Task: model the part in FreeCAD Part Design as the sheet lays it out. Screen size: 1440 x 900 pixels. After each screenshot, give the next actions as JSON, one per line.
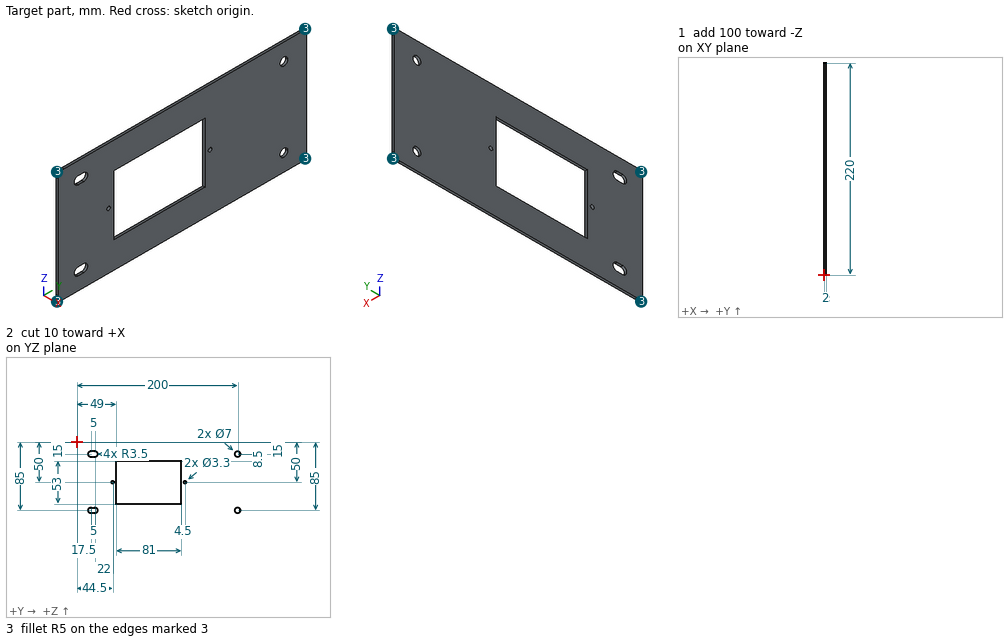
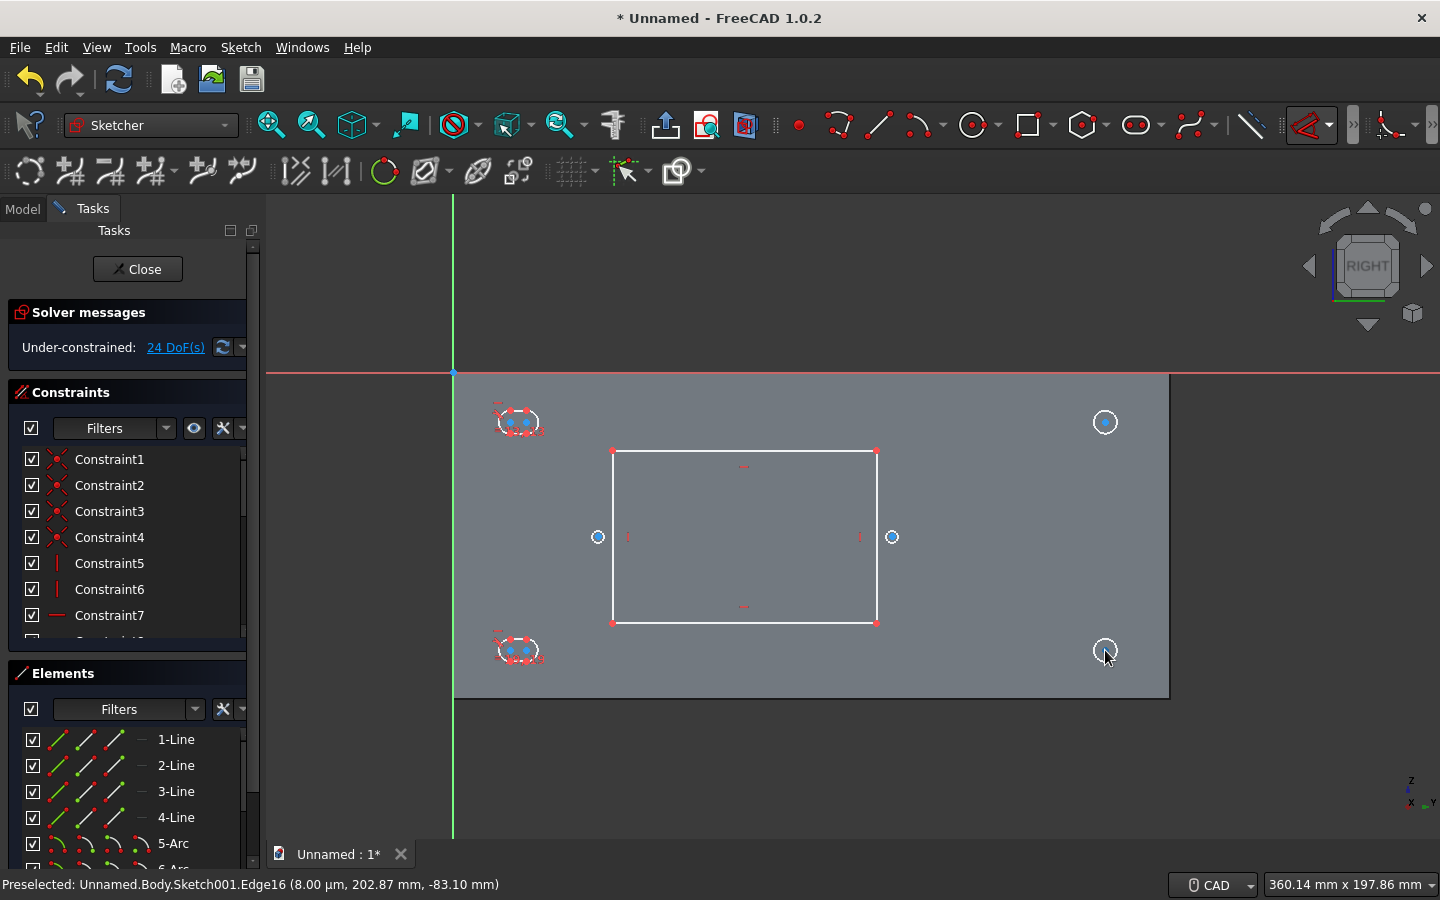
{"action": "scroll", "coordinate": [501, 415], "scroll_direction": "up", "scroll_amount": 2}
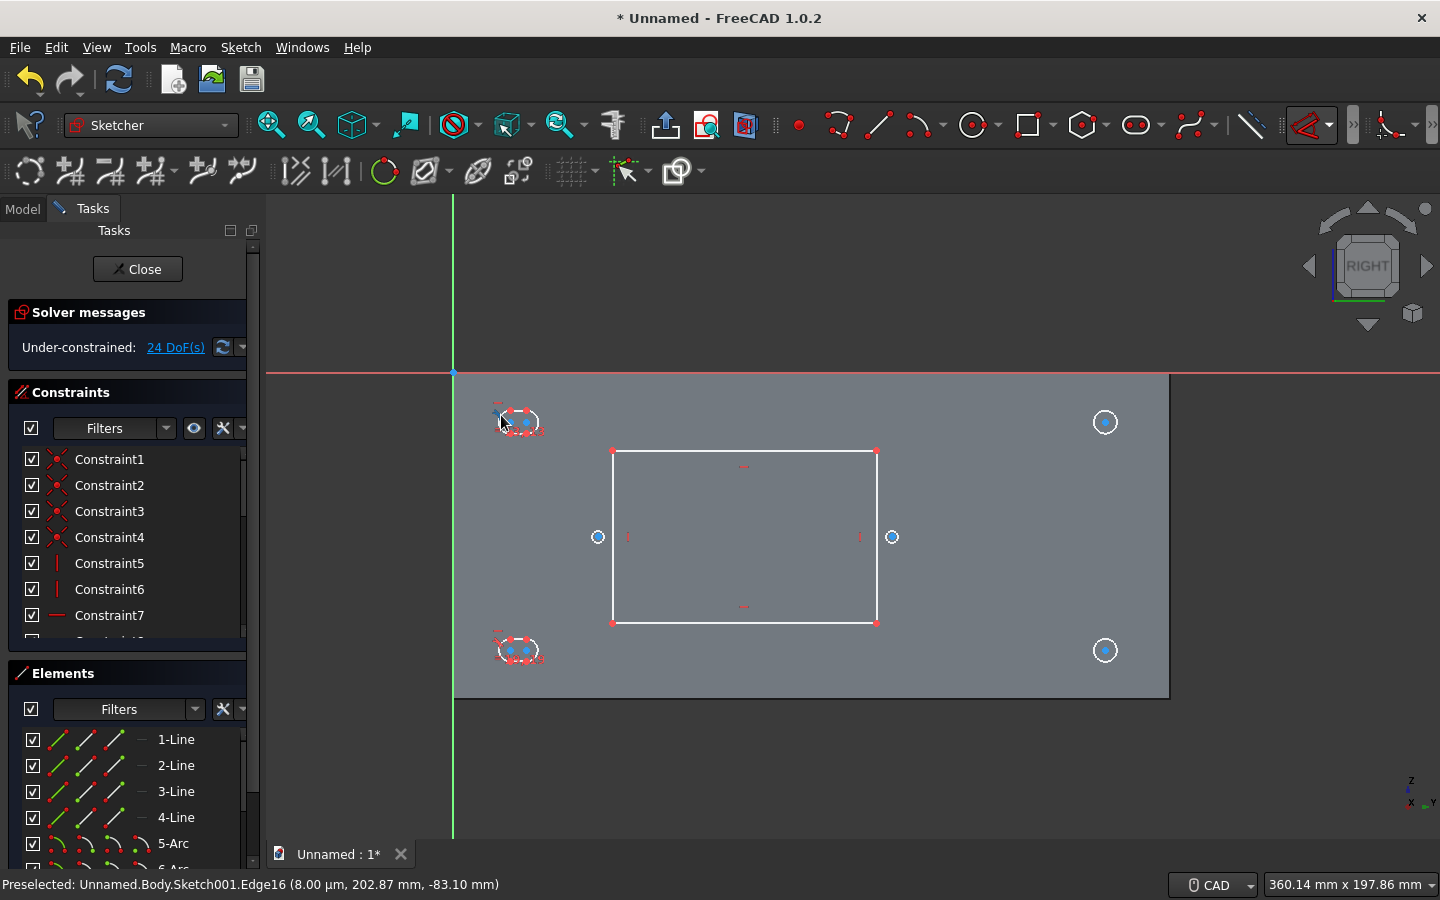
{"action": "left_click", "coordinate": [501, 415]}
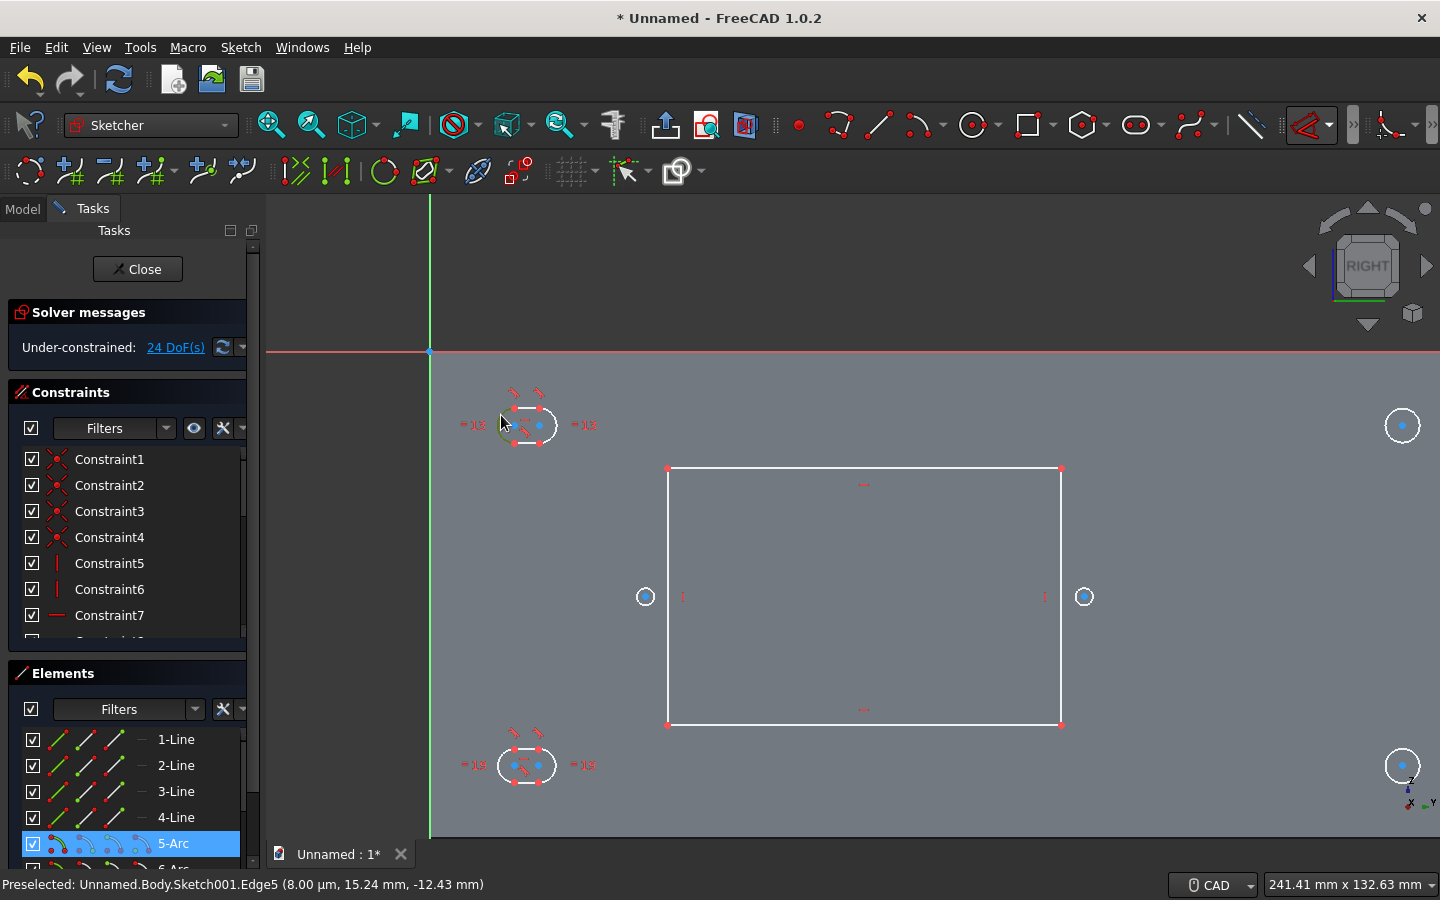
{"action": "left_click", "coordinate": [501, 756]}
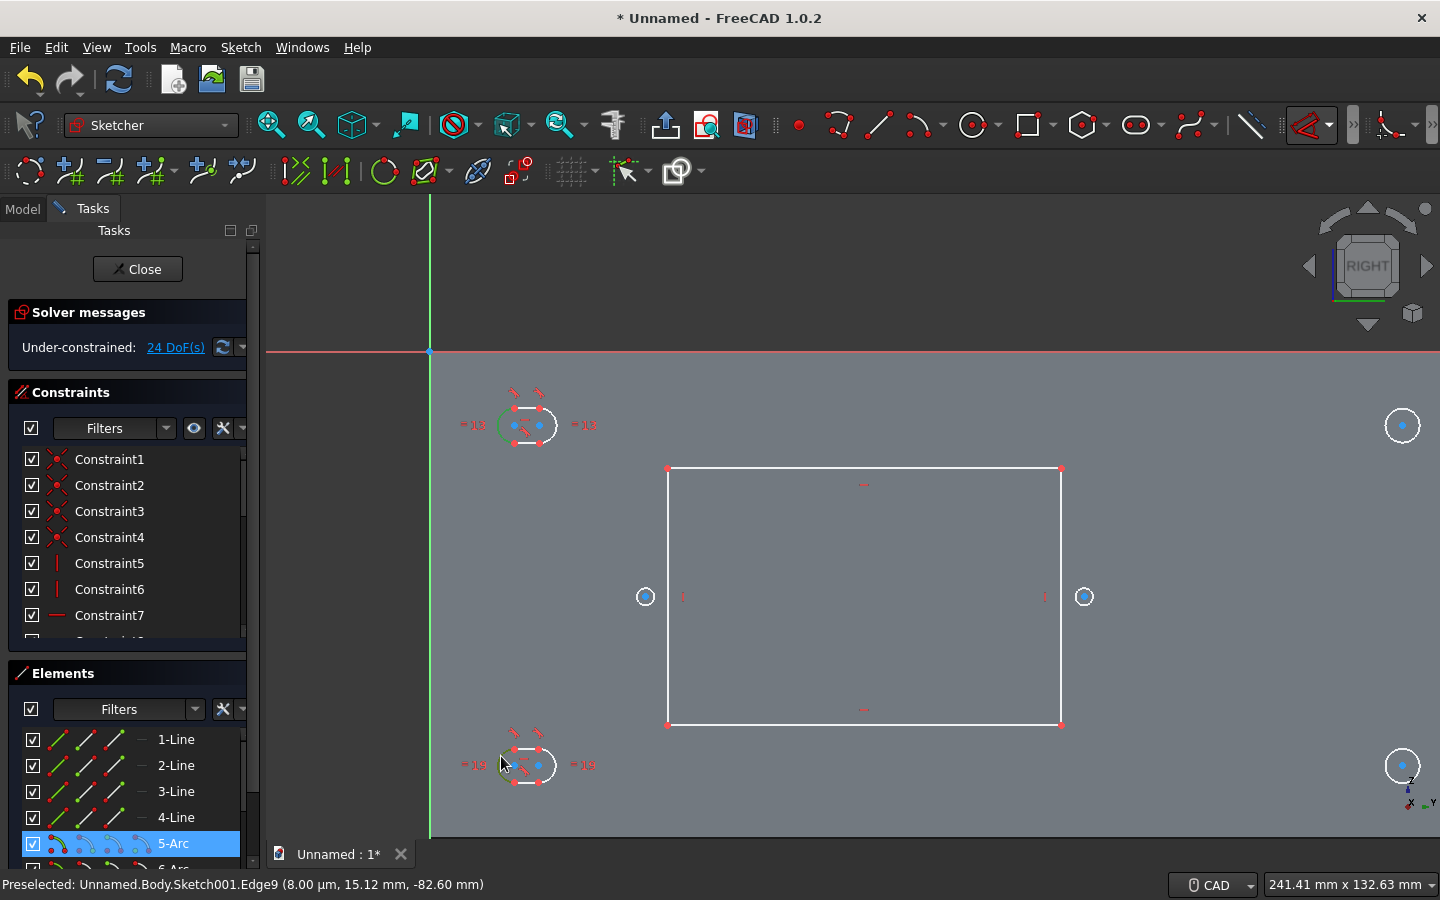
{"action": "key", "text": "e"}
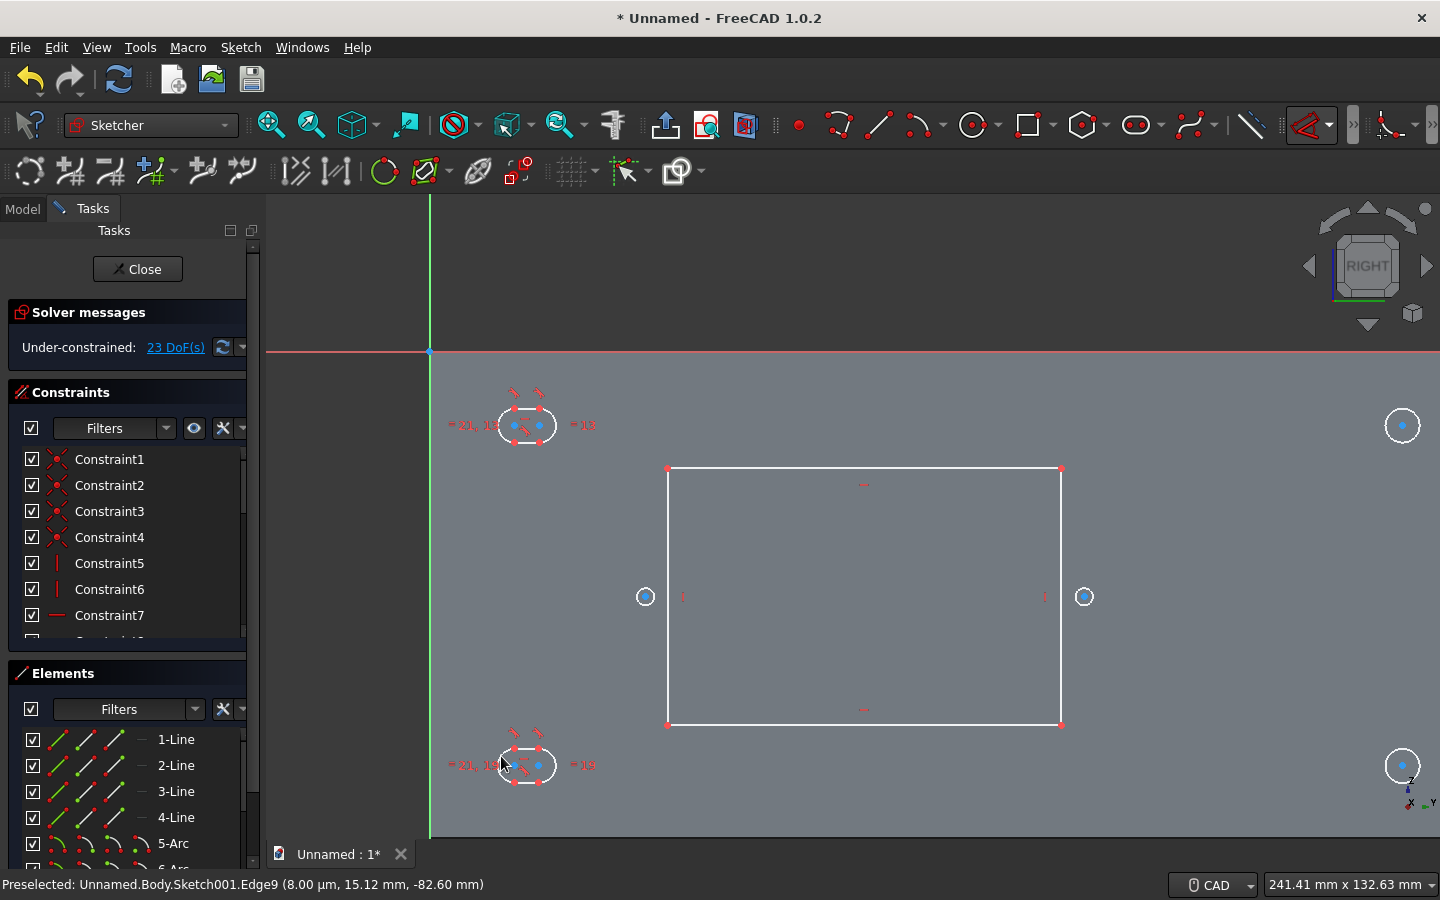
{"action": "scroll", "coordinate": [646, 588], "scroll_direction": "up", "scroll_amount": 3}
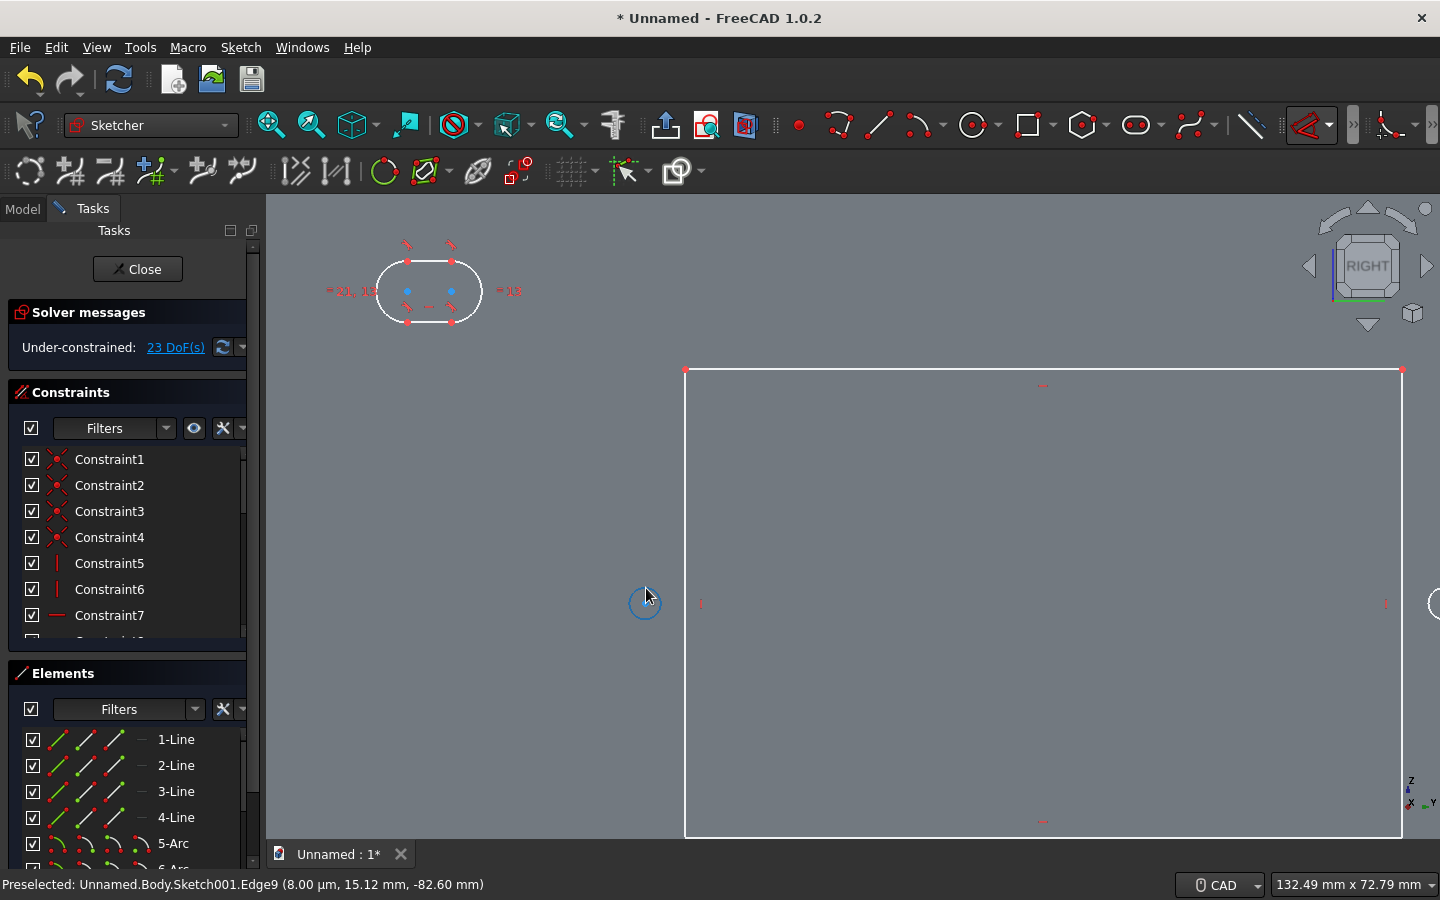
{"action": "left_click", "coordinate": [645, 588]}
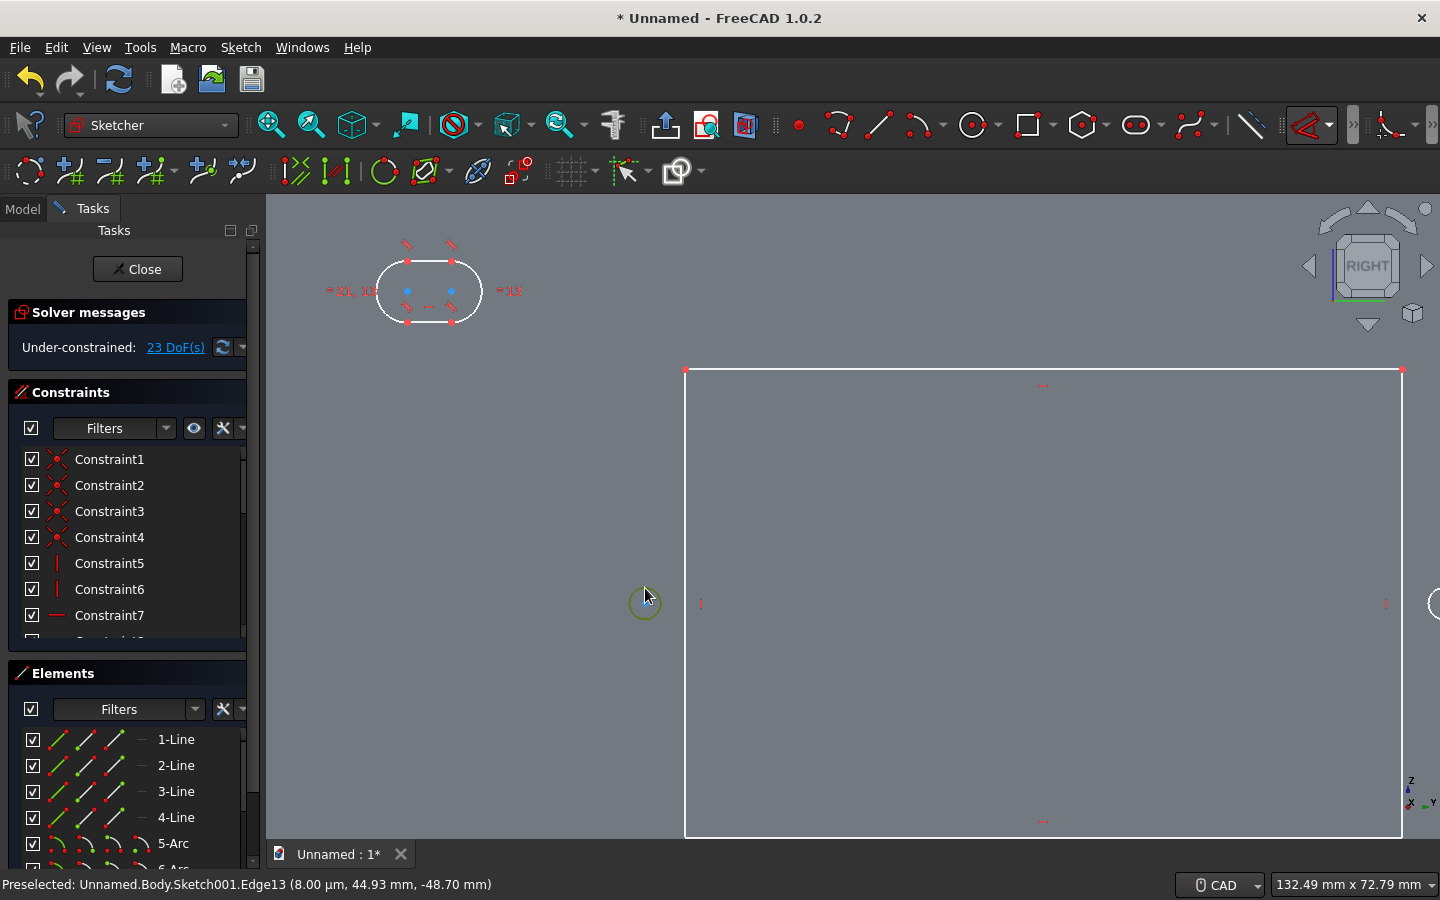
{"action": "scroll", "coordinate": [570, 497], "scroll_direction": "down", "scroll_amount": 5}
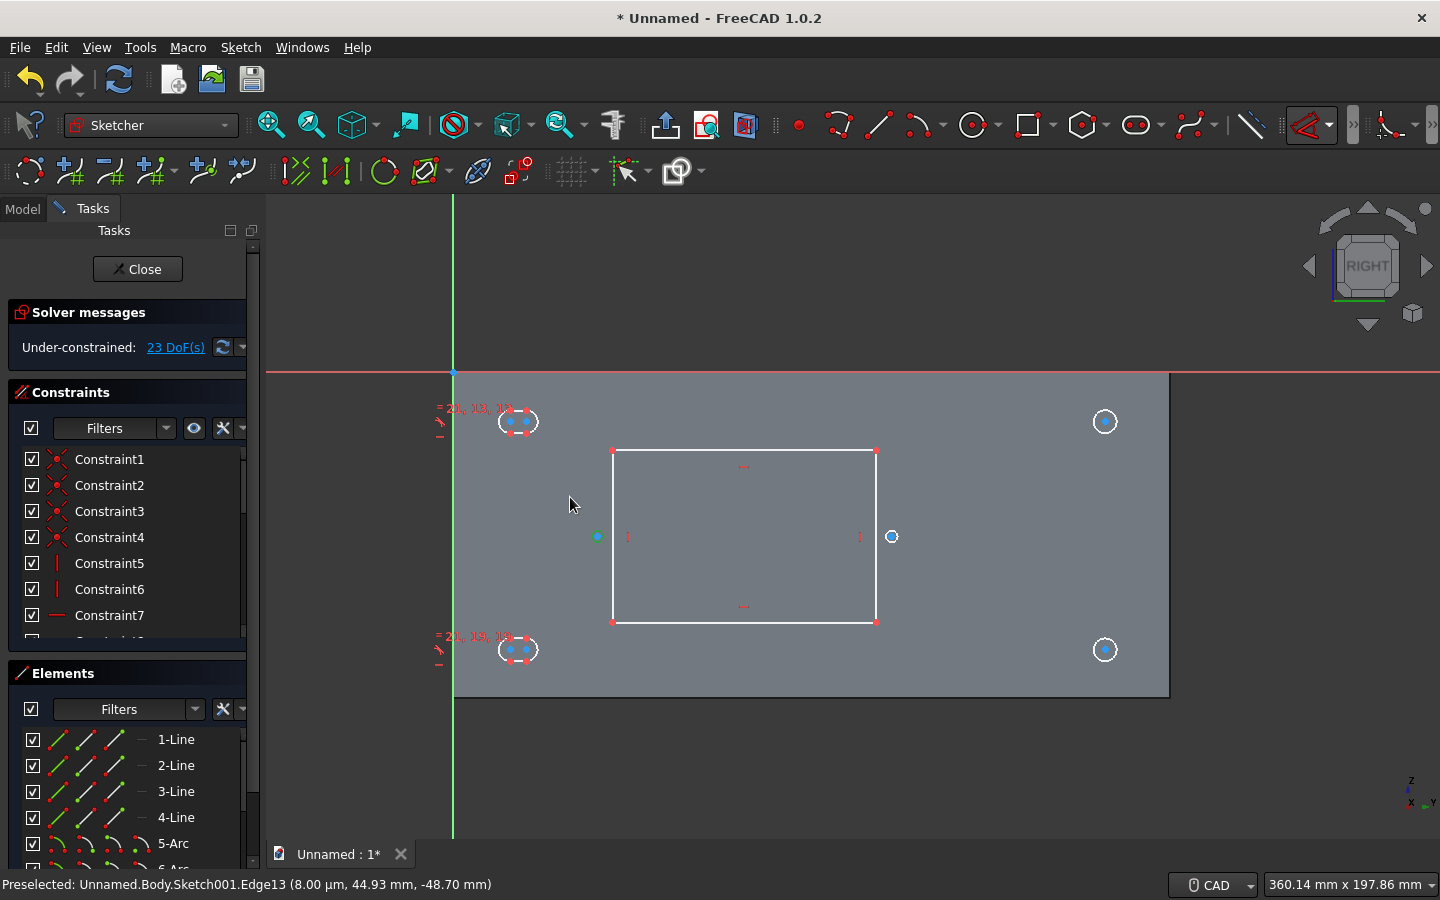
{"action": "scroll", "coordinate": [896, 532], "scroll_direction": "up", "scroll_amount": 5}